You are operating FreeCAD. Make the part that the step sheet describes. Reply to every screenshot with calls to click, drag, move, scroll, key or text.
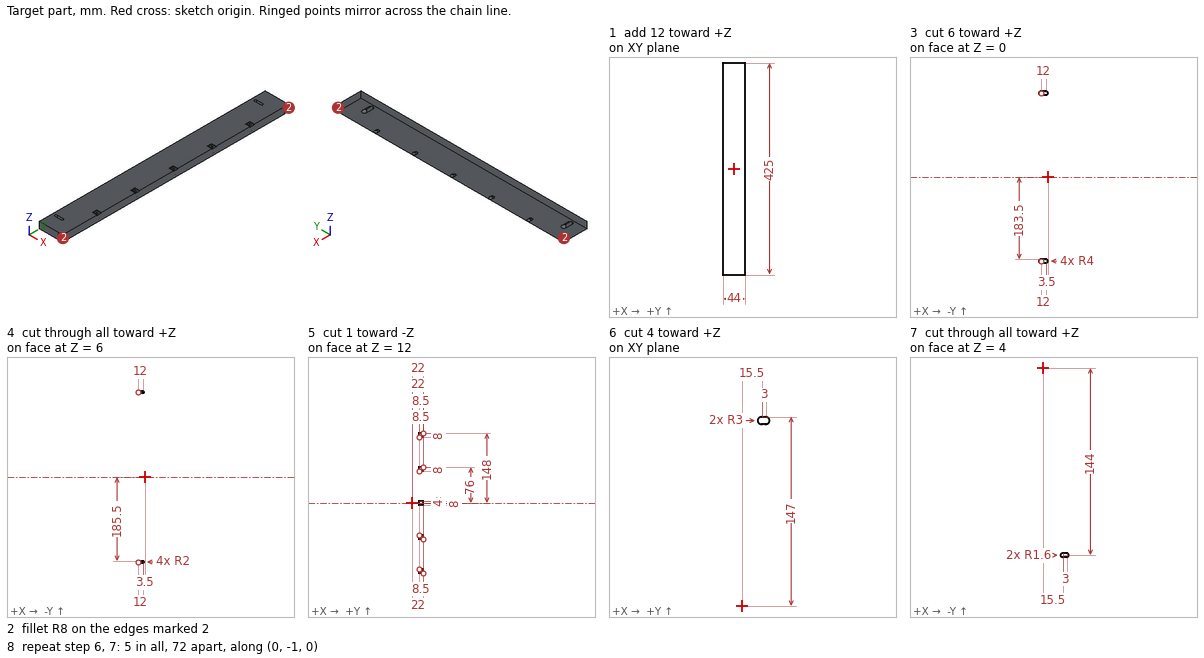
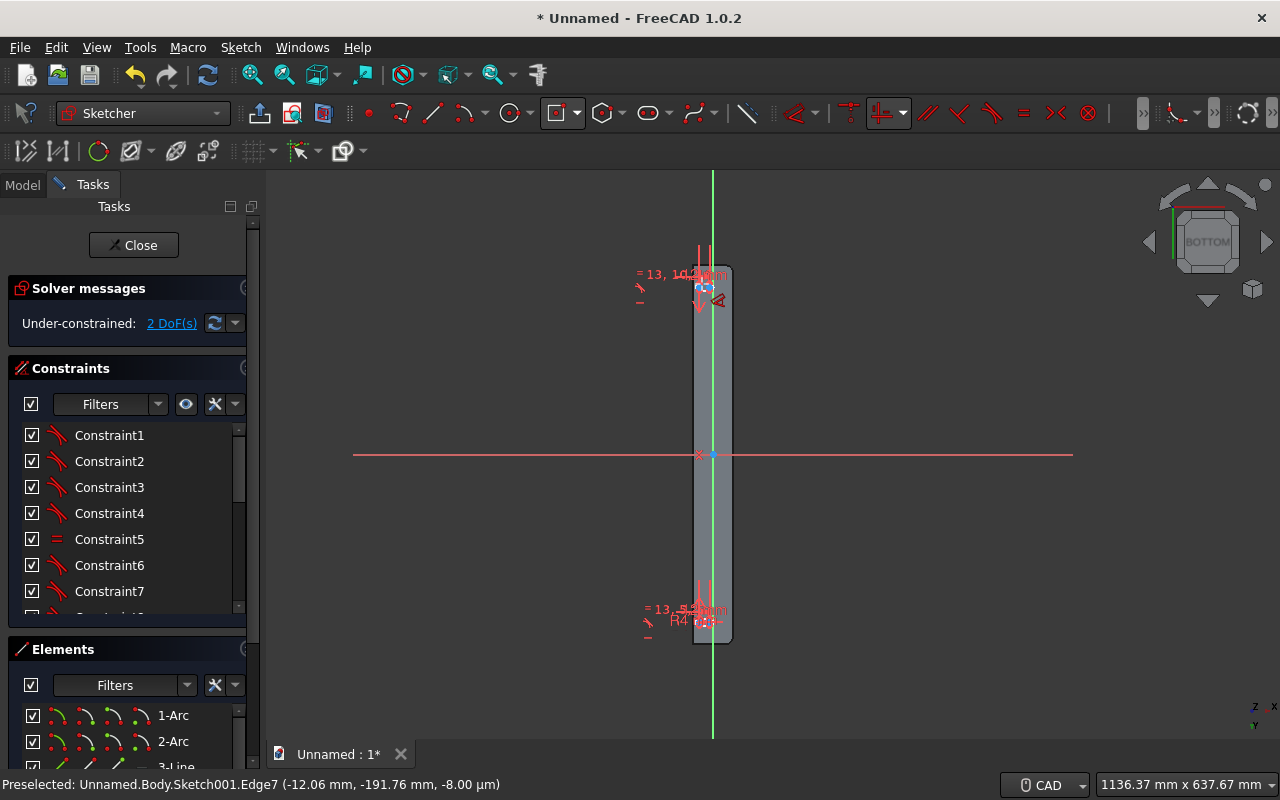
scroll(710, 626, up, 13)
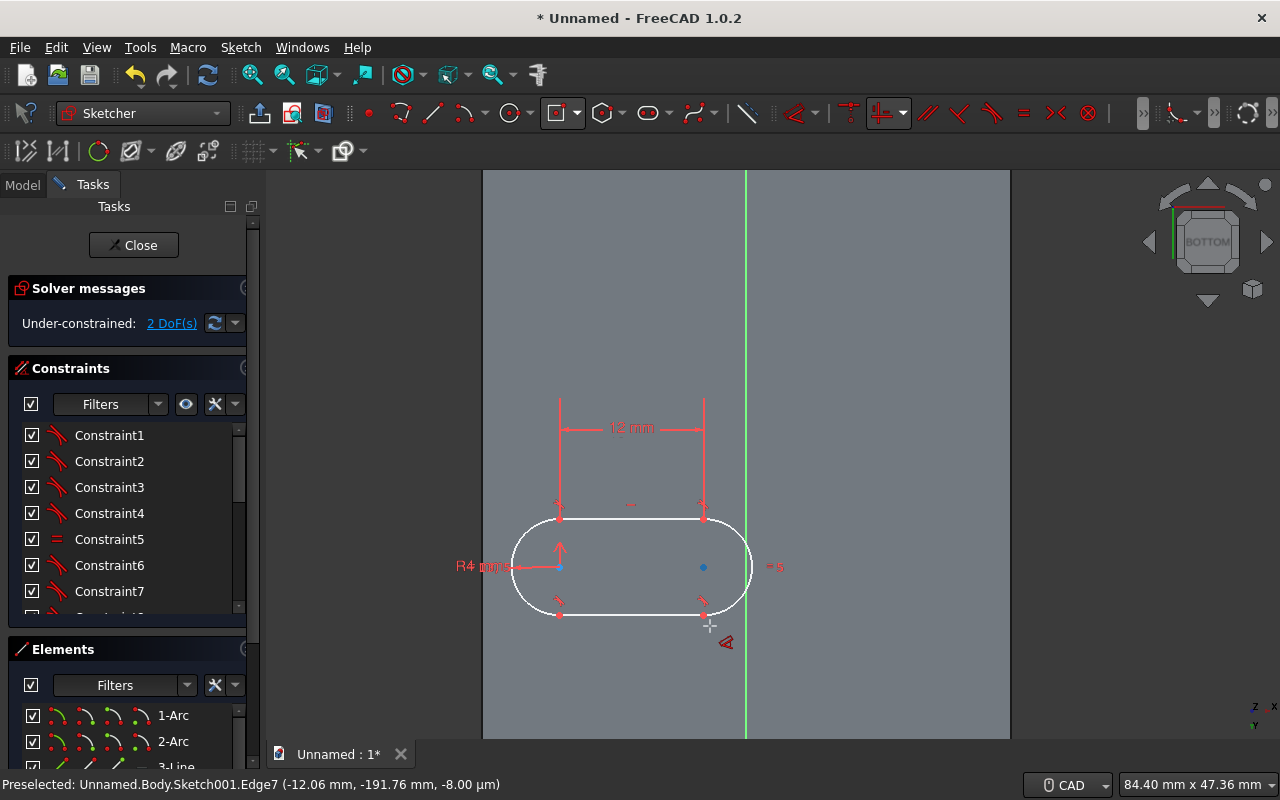
click(704, 615)
click(725, 649)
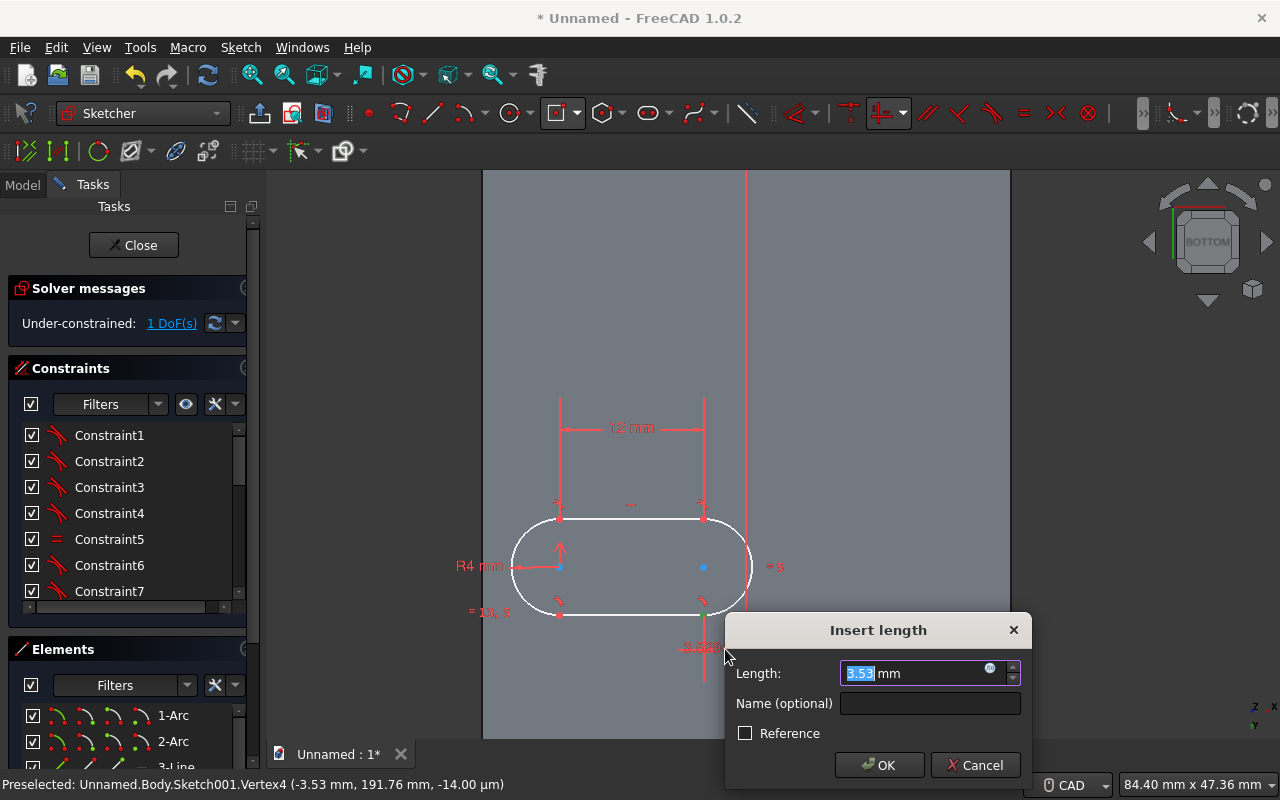
text(3.5)
key(Return)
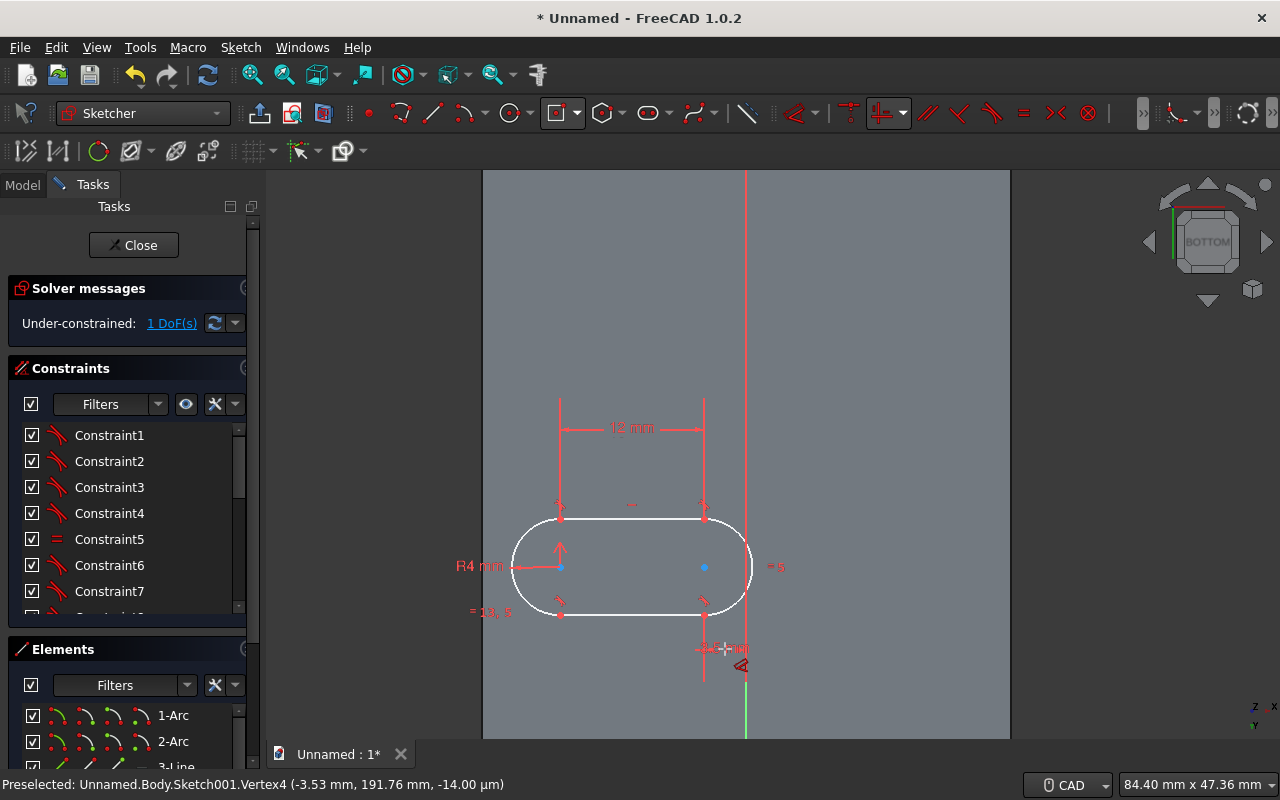
scroll(710, 626, down, 13)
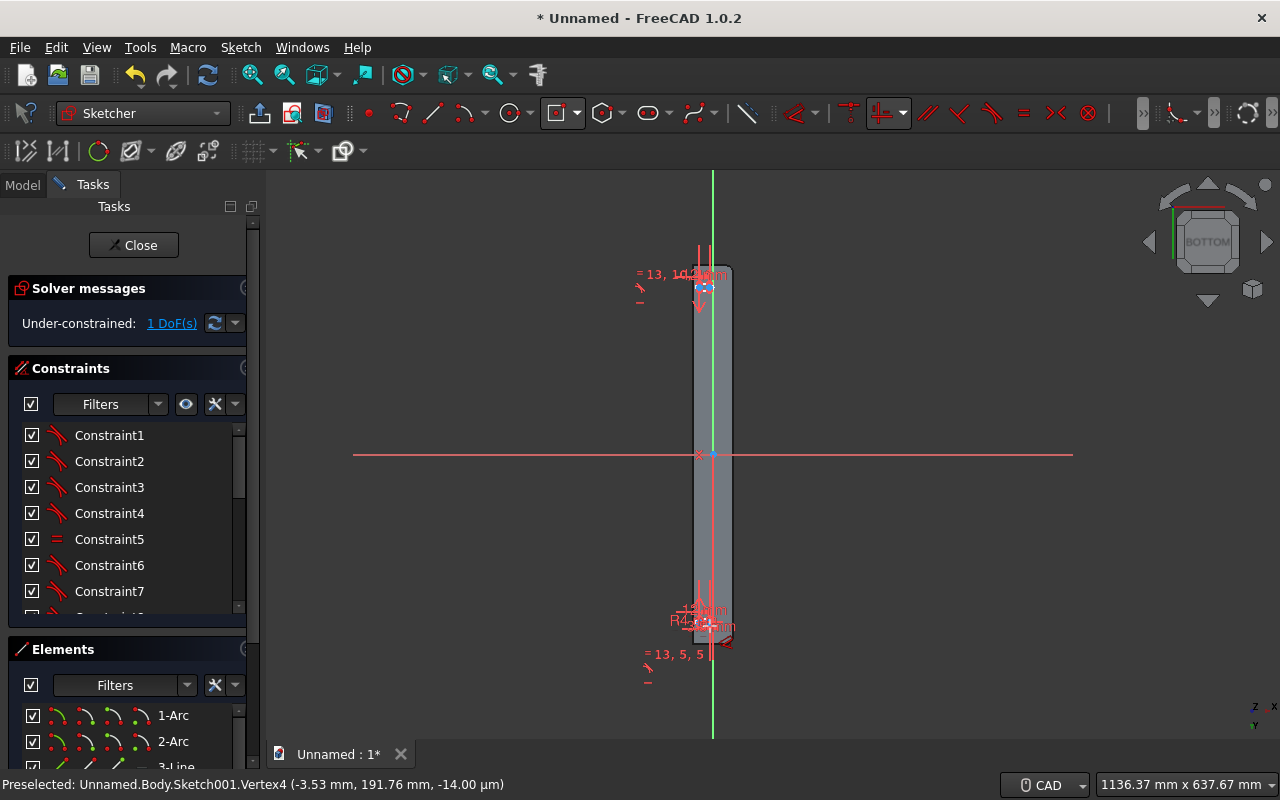
scroll(699, 619, up, 7)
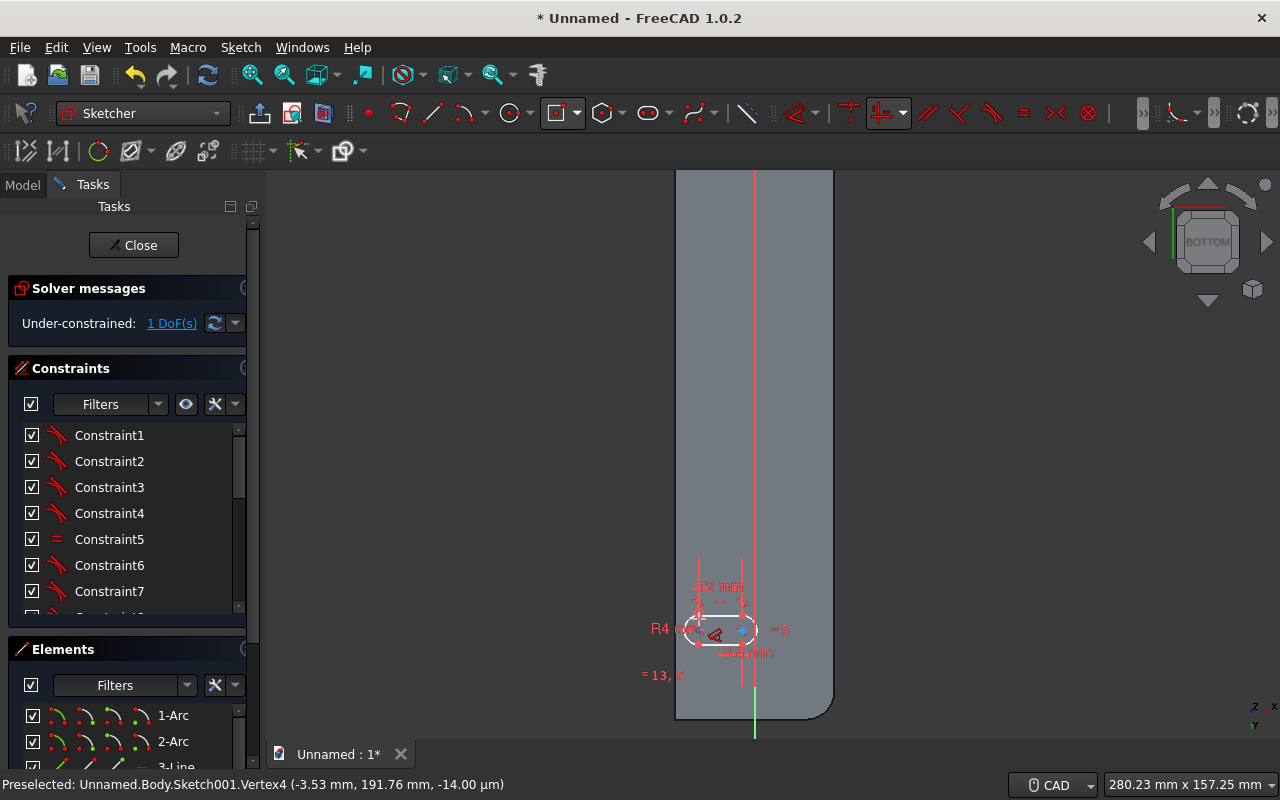
click(699, 616)
click(789, 407)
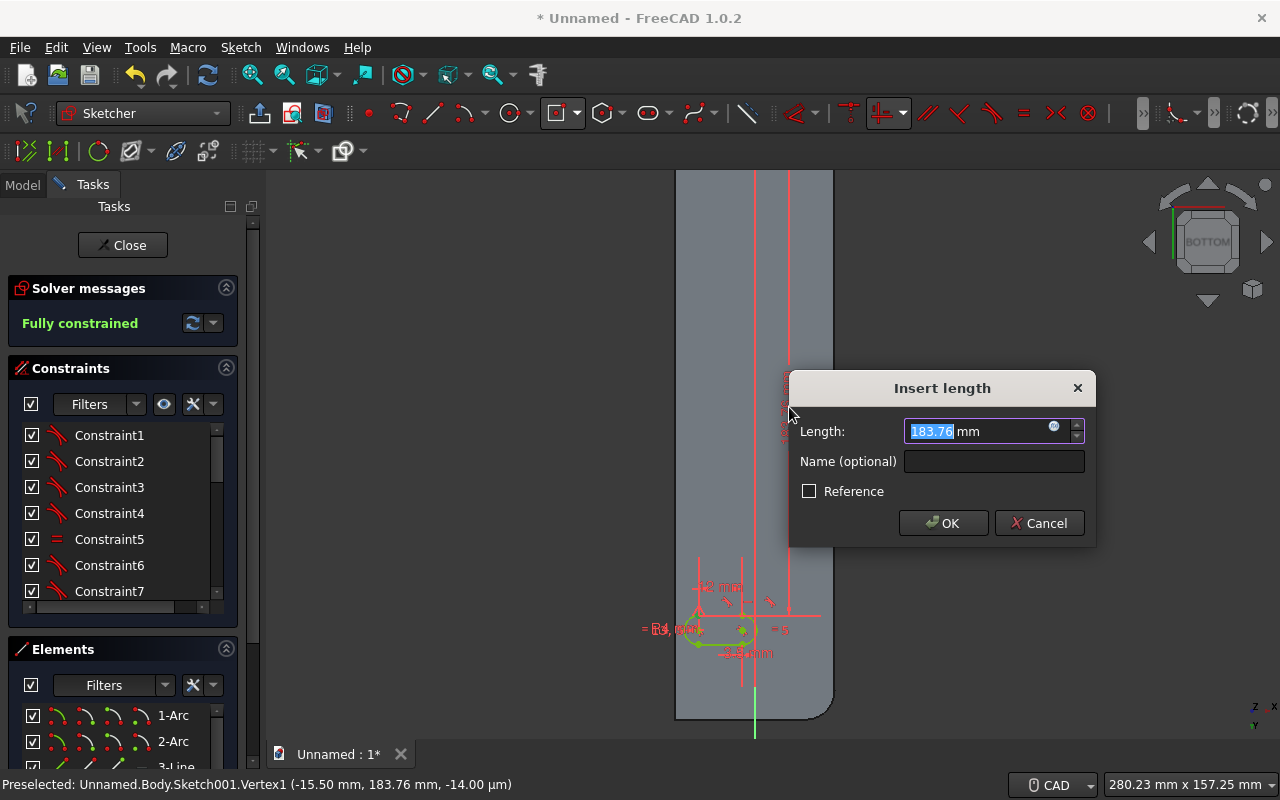
text(183.5)
key(Return)
key(Escape)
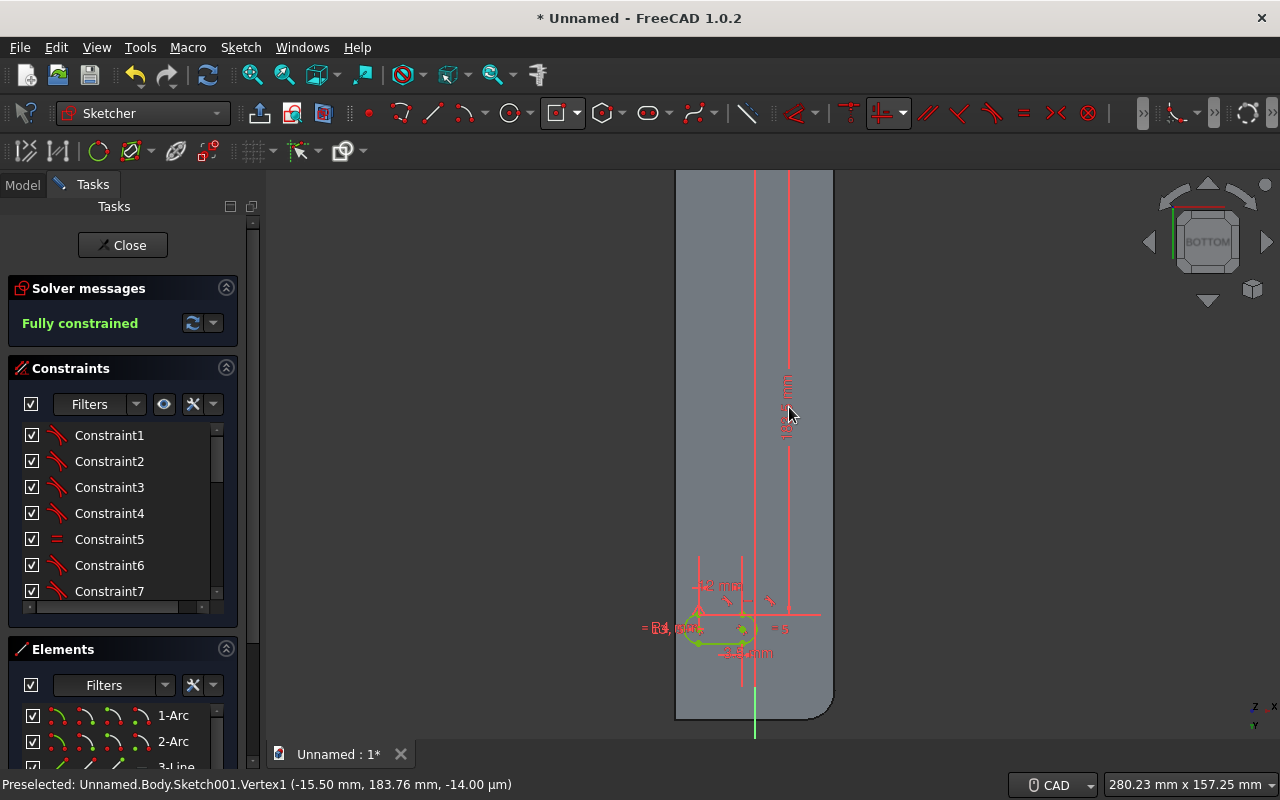
click(123, 245)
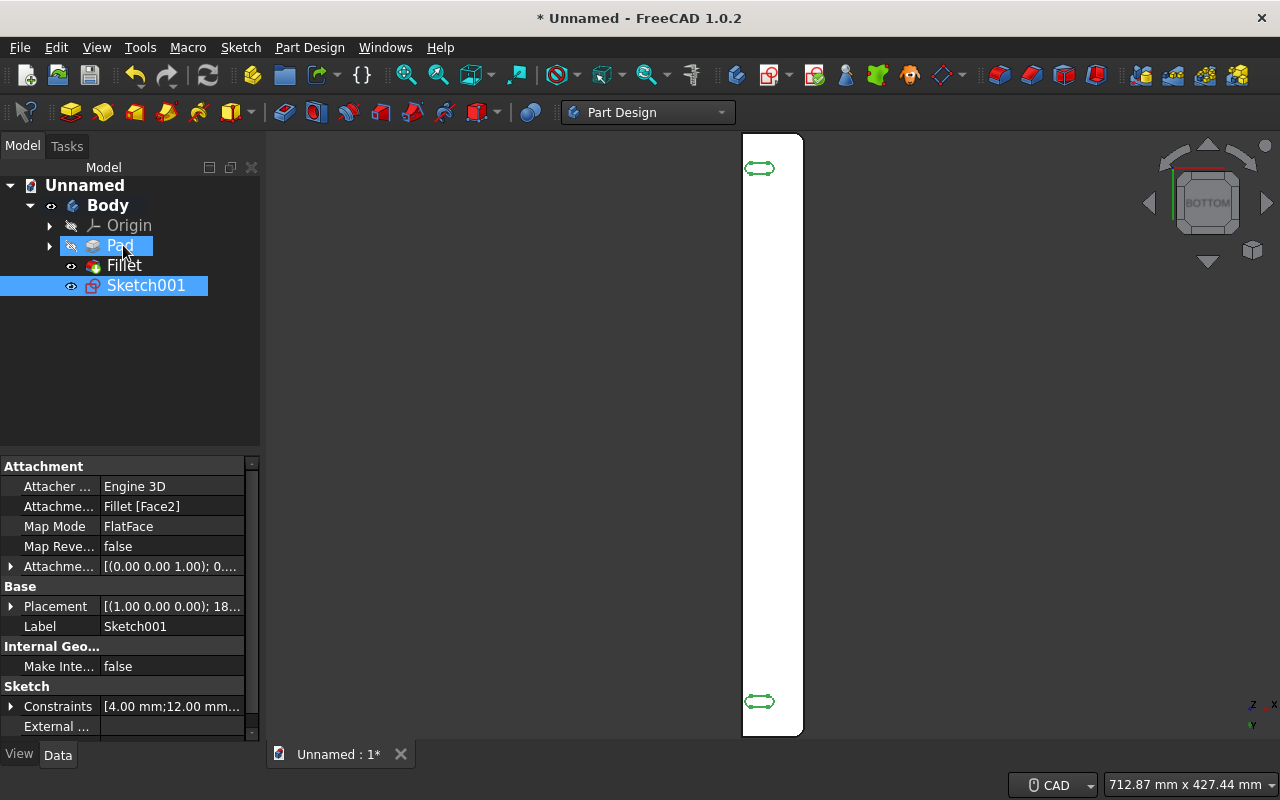
click(286, 112)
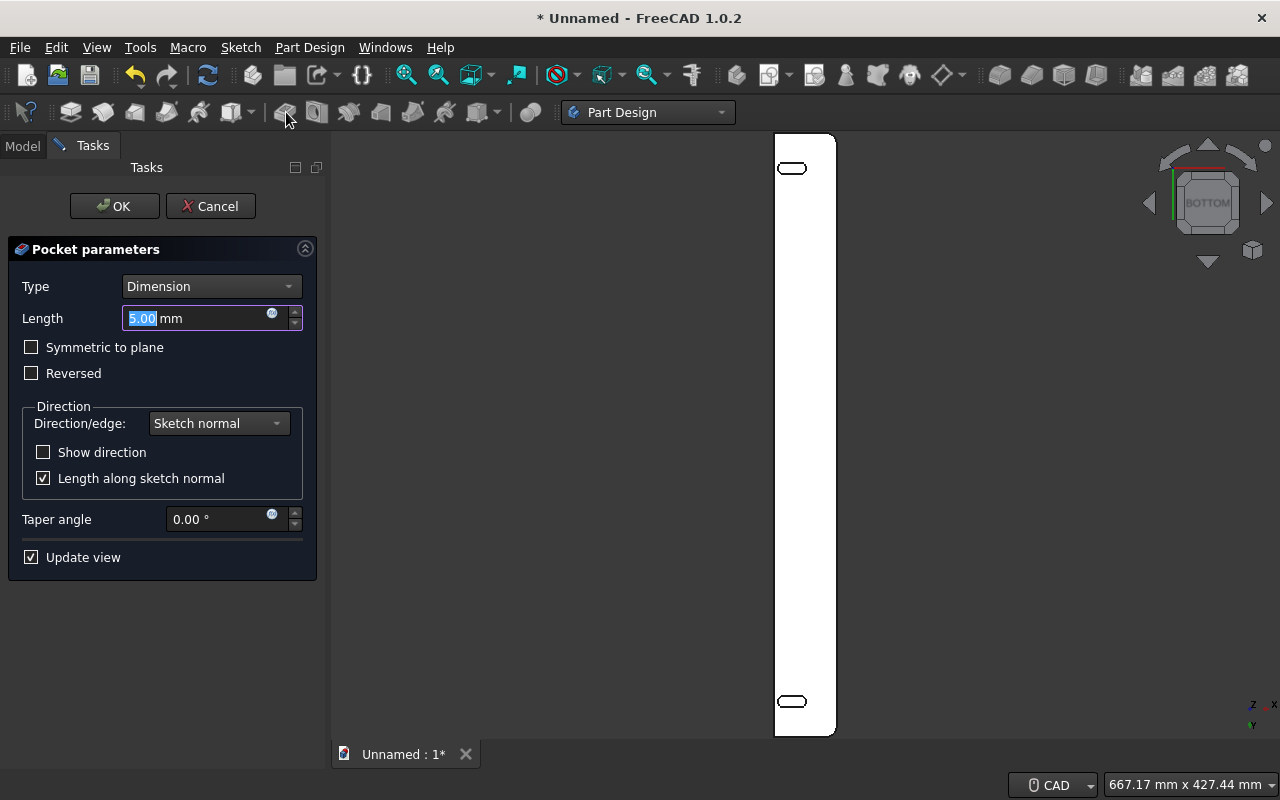
text(6)
key(Tab)